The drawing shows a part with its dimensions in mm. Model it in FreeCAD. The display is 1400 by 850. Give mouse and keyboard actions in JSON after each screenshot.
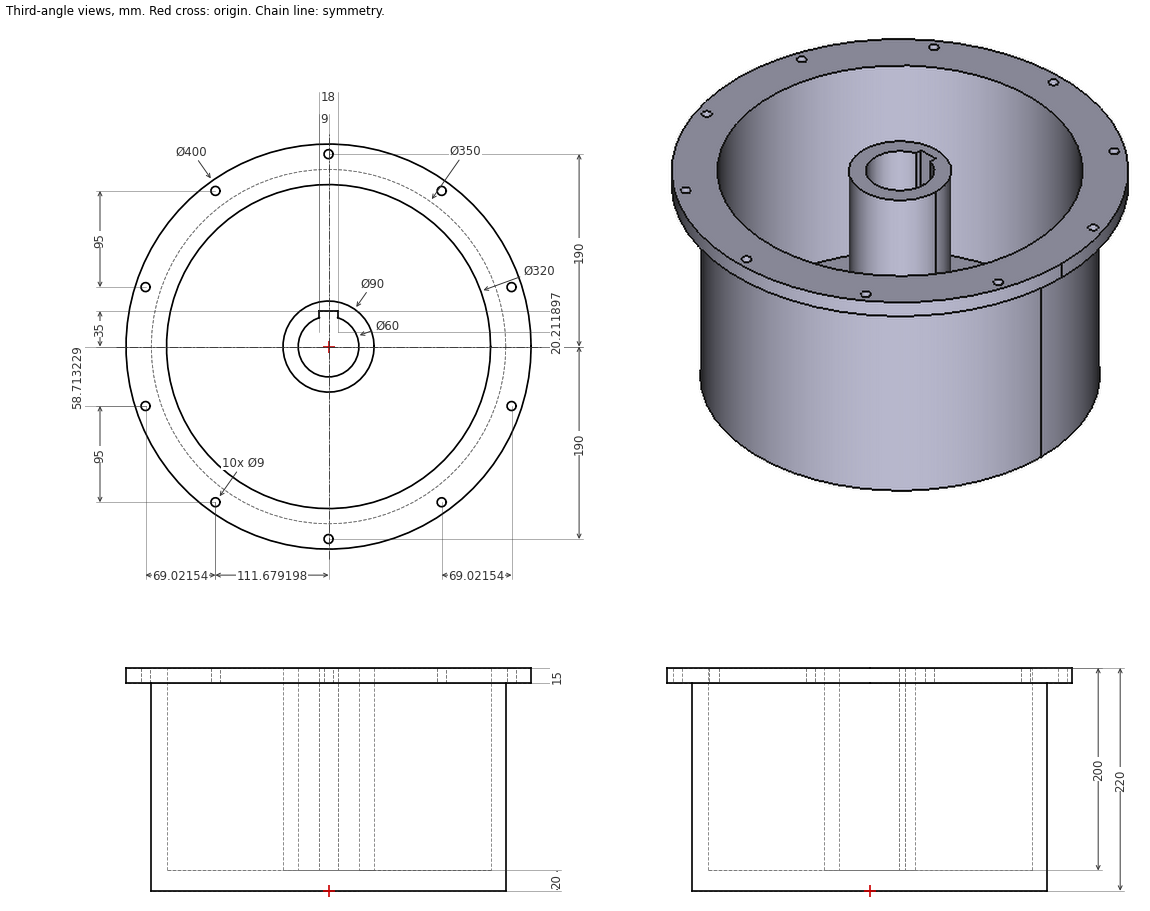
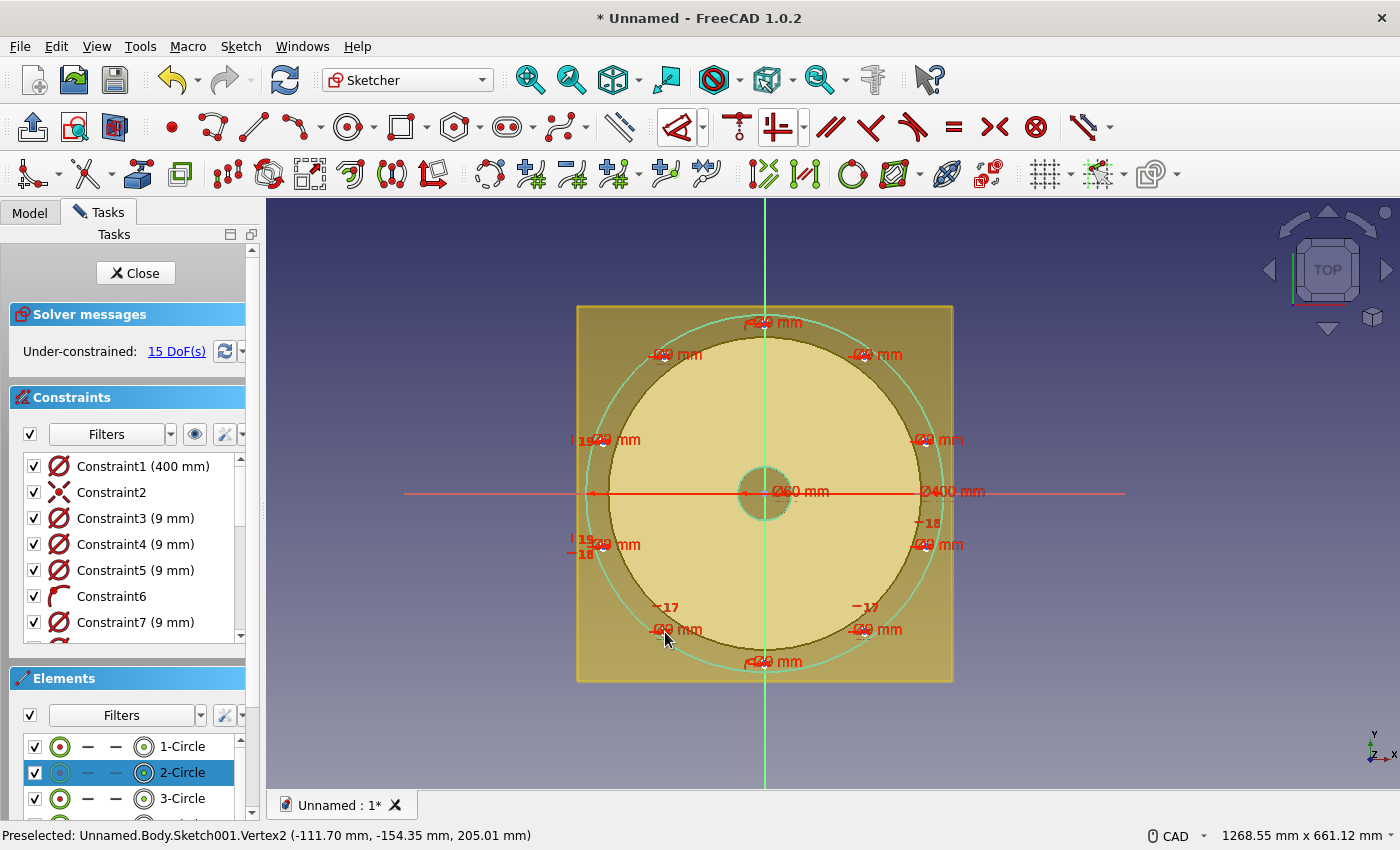
{"action": "left_click", "coordinate": [665, 357]}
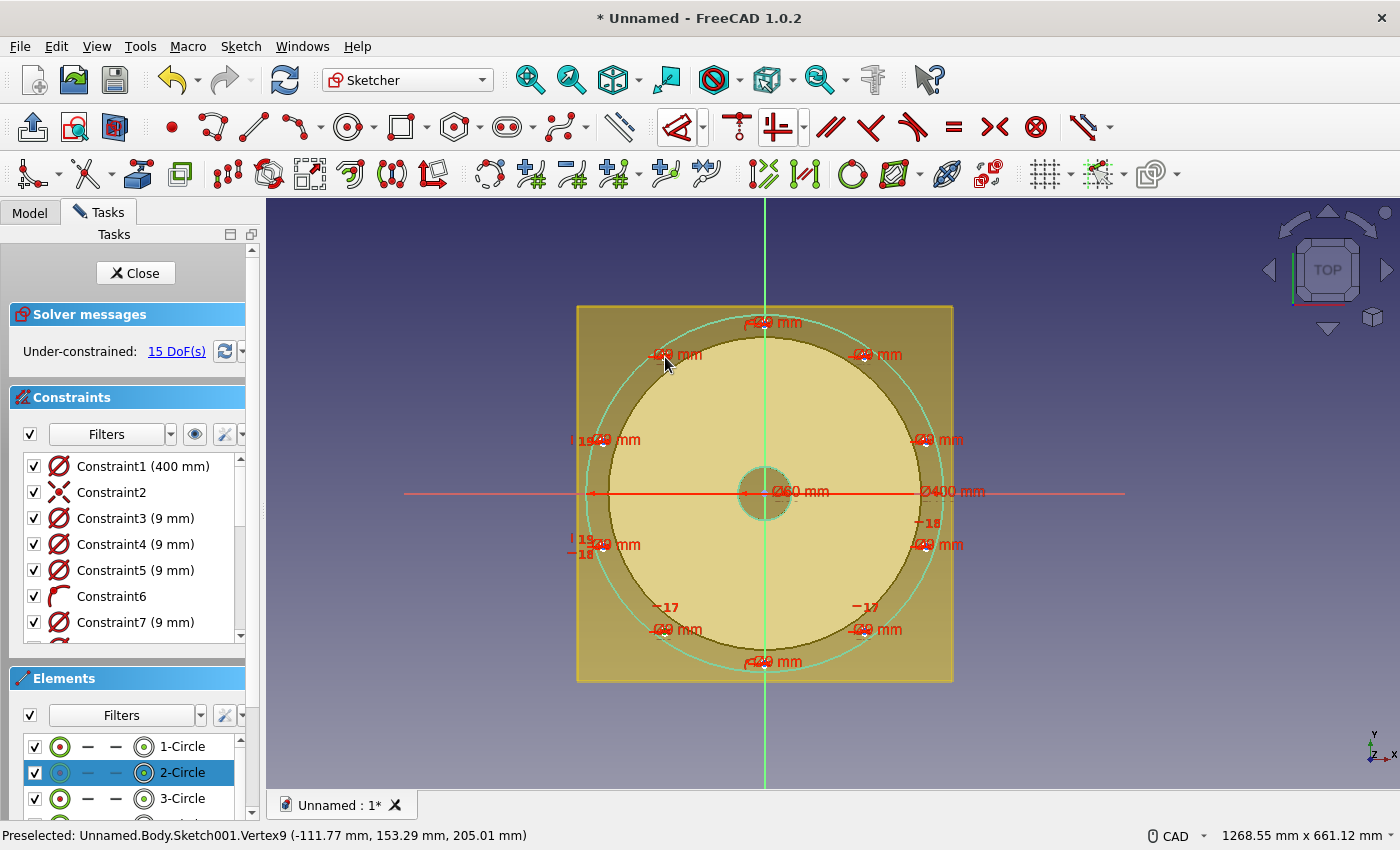
{"action": "key", "text": "v"}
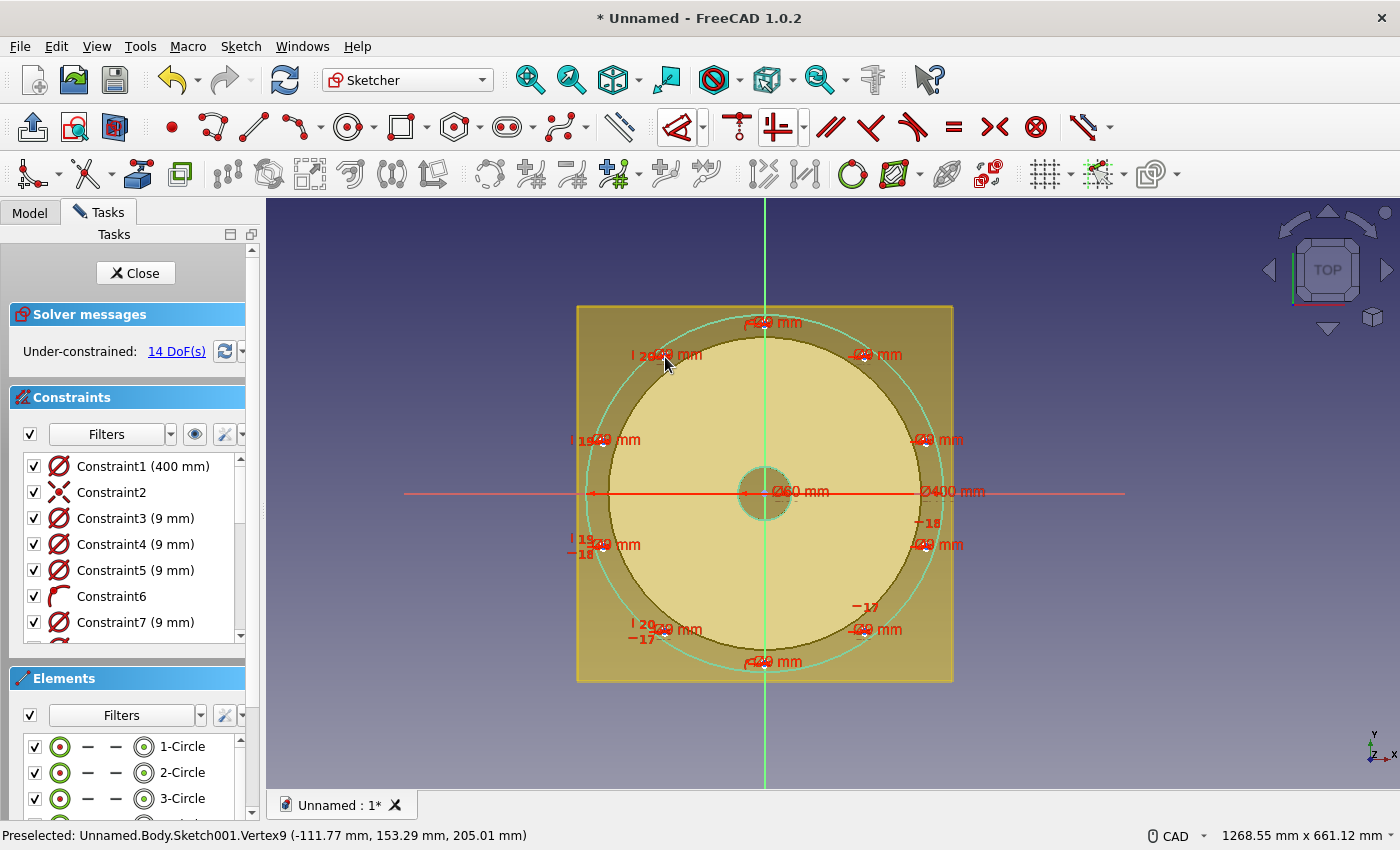
{"action": "left_click", "coordinate": [926, 547]}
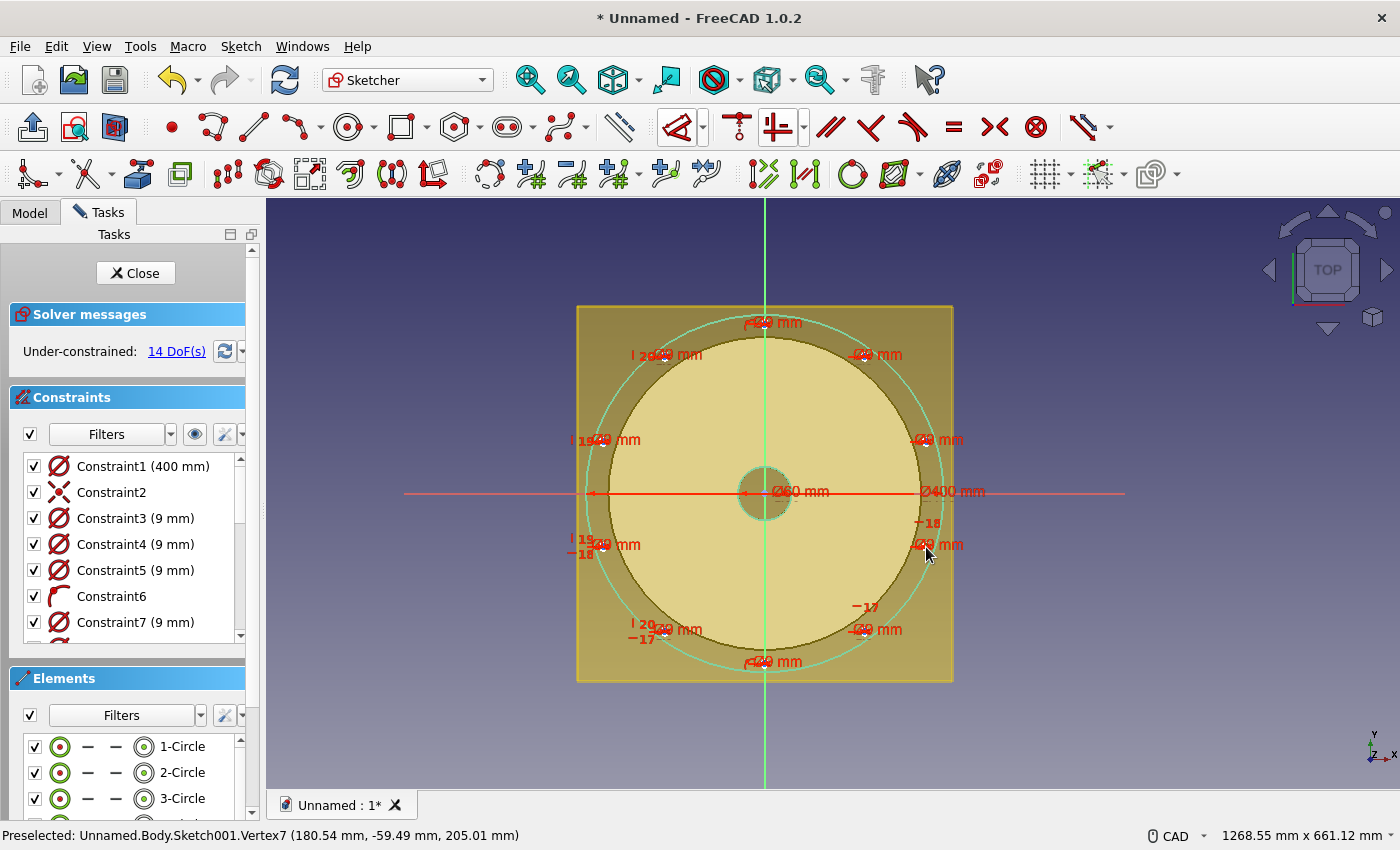
{"action": "left_click", "coordinate": [926, 442]}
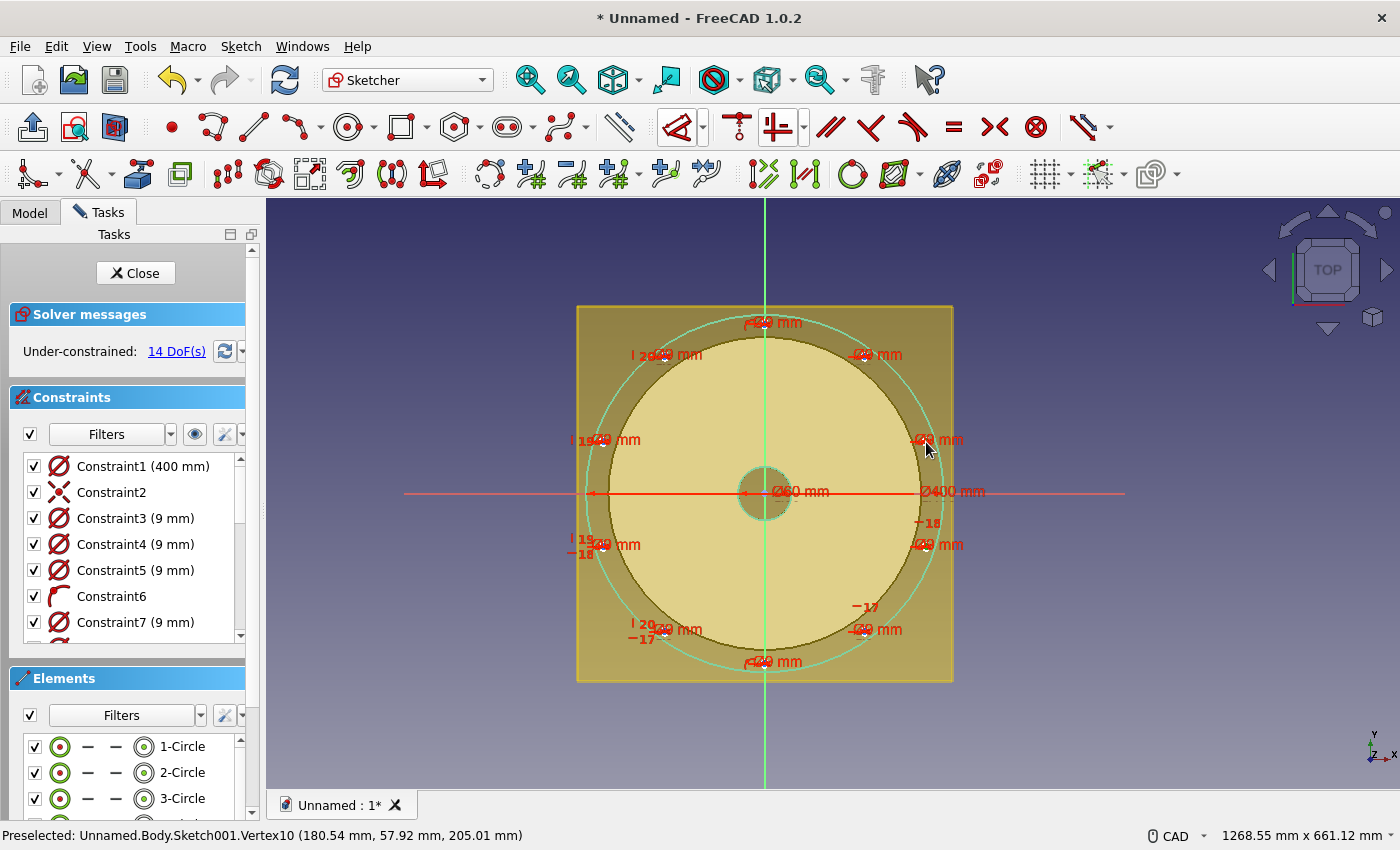
{"action": "key", "text": "v"}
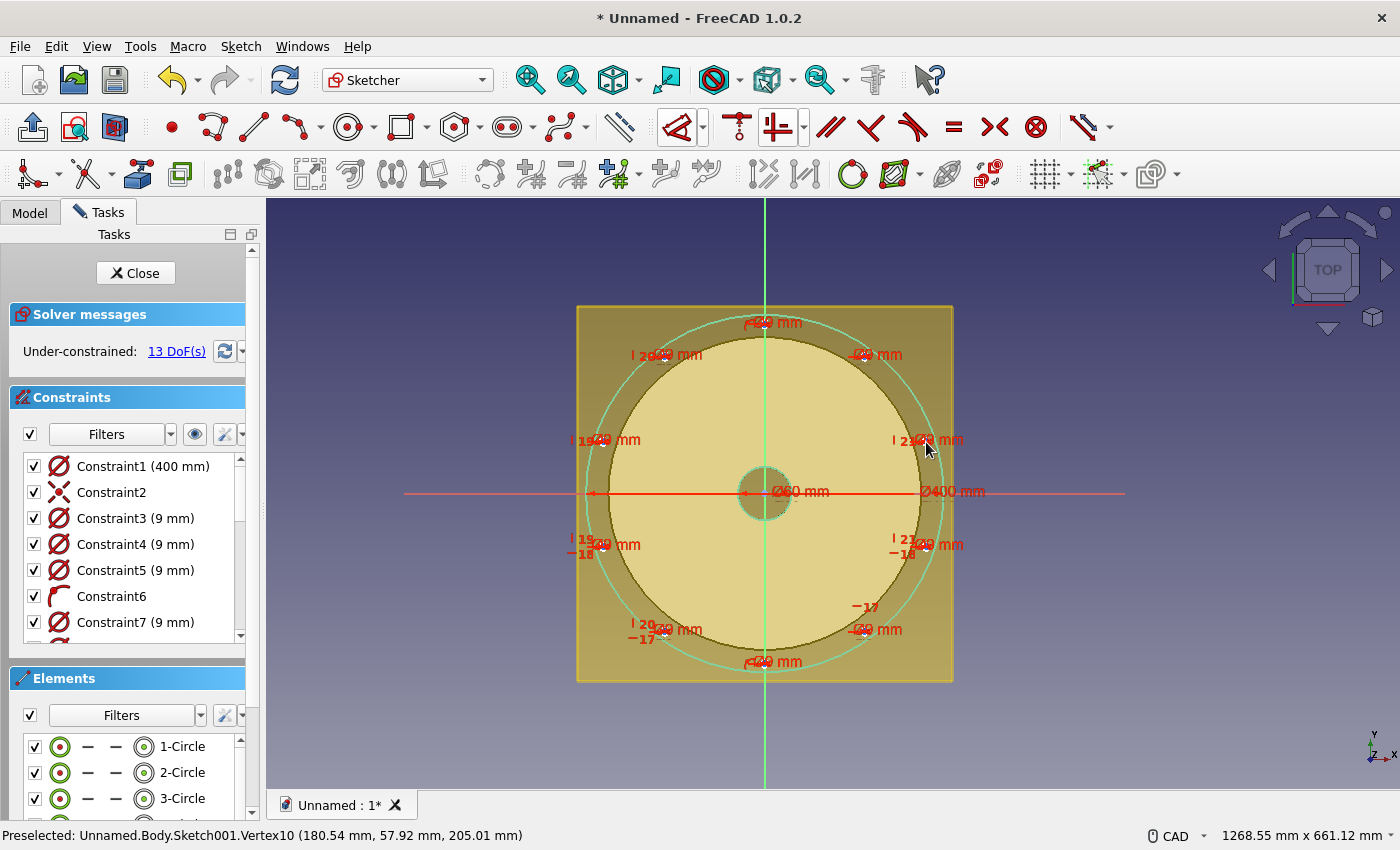
{"action": "left_click", "coordinate": [665, 357]}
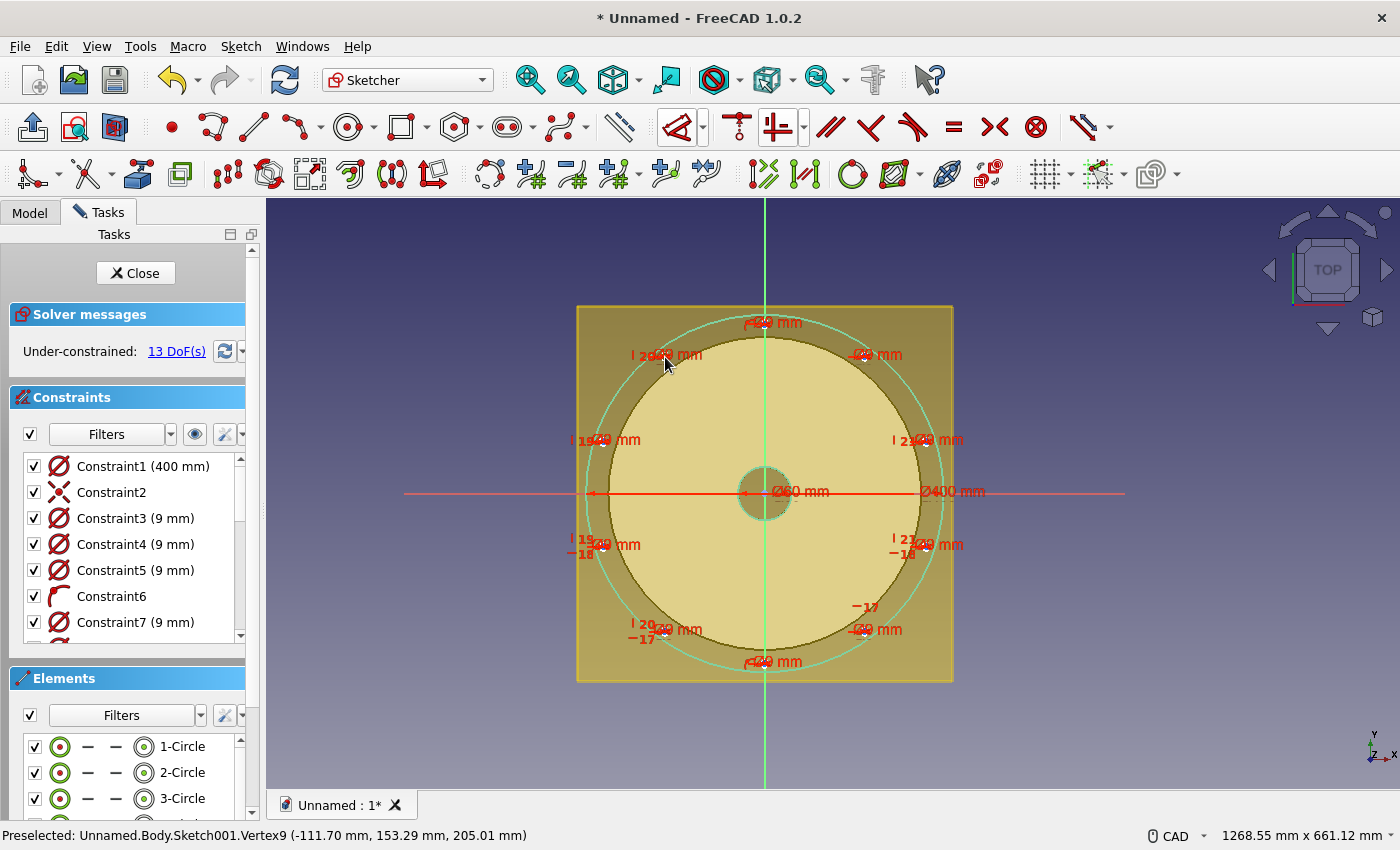
{"action": "left_click", "coordinate": [865, 357]}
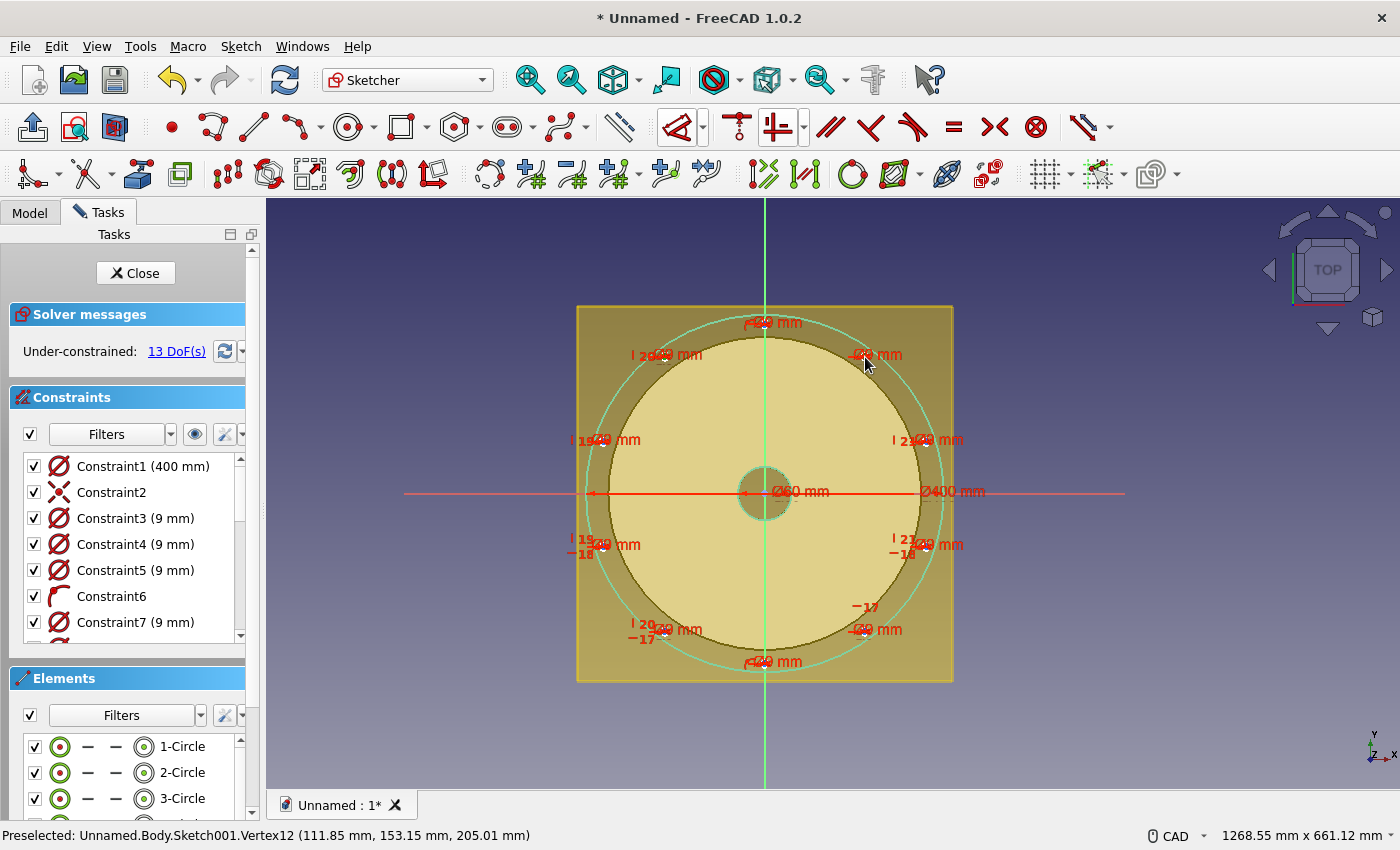
{"action": "left_click", "coordinate": [804, 128]}